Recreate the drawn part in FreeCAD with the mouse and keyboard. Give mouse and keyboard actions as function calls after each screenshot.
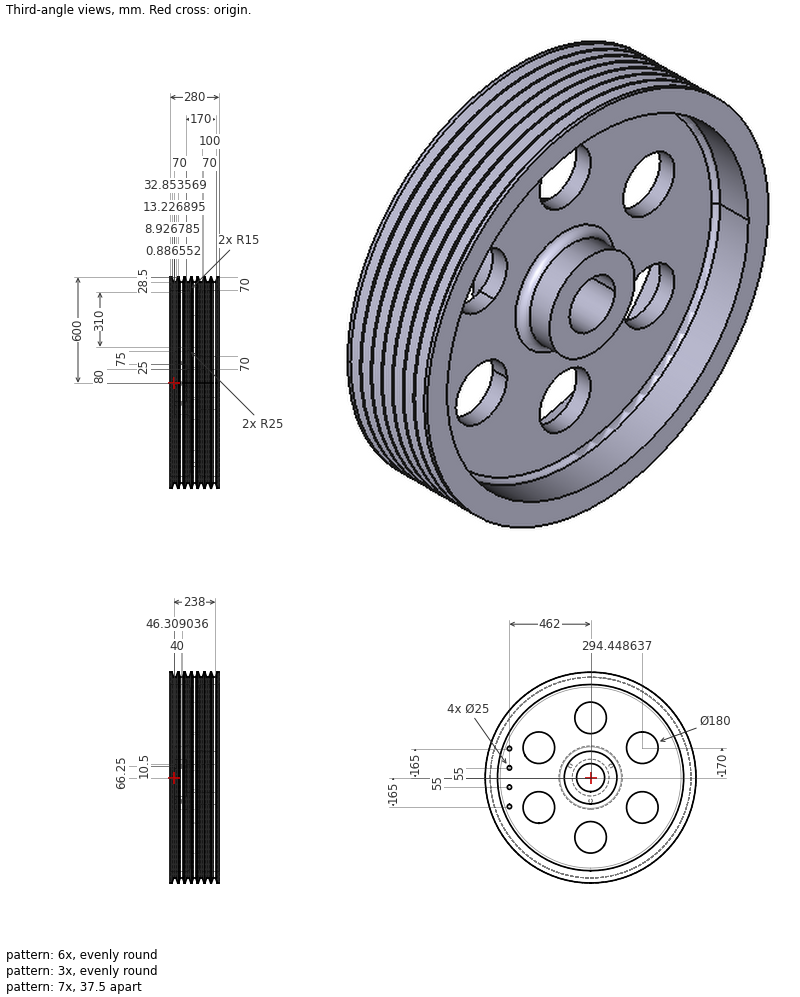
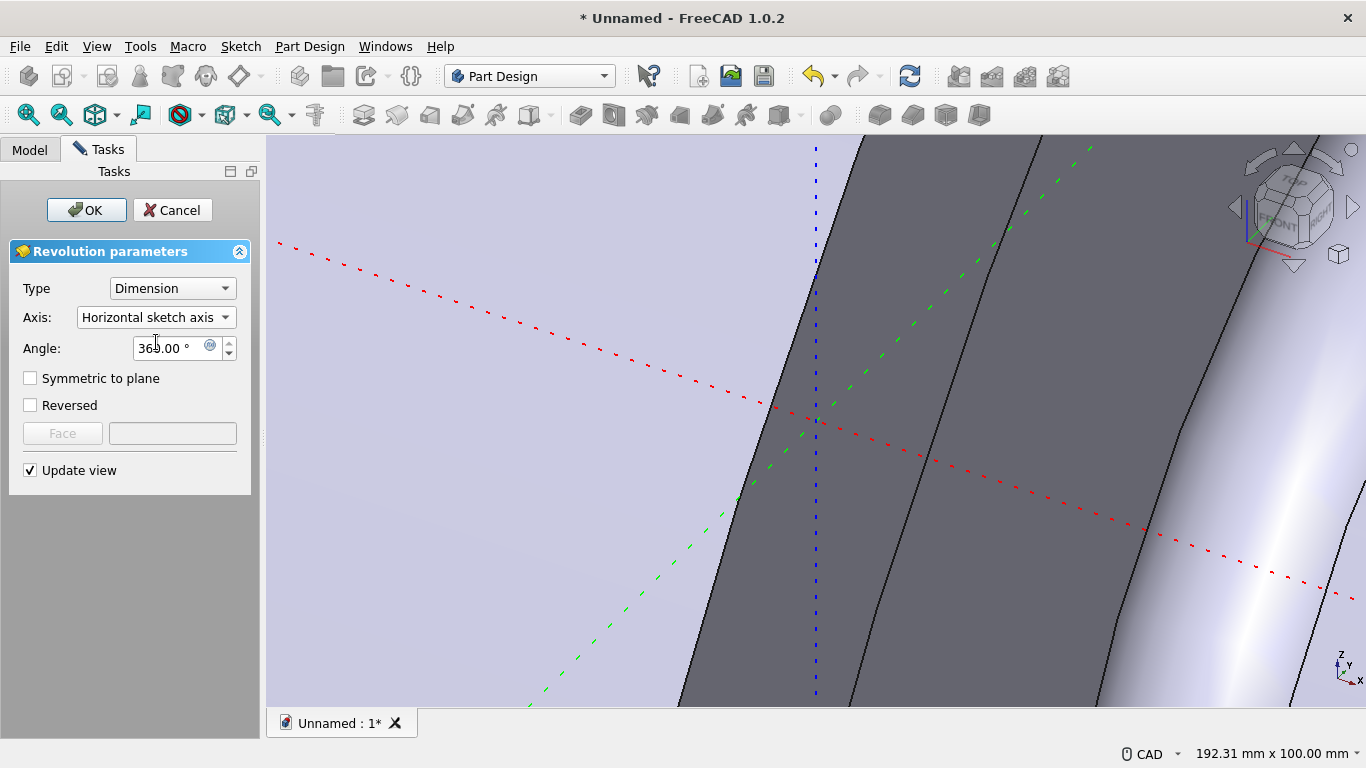
click(87, 210)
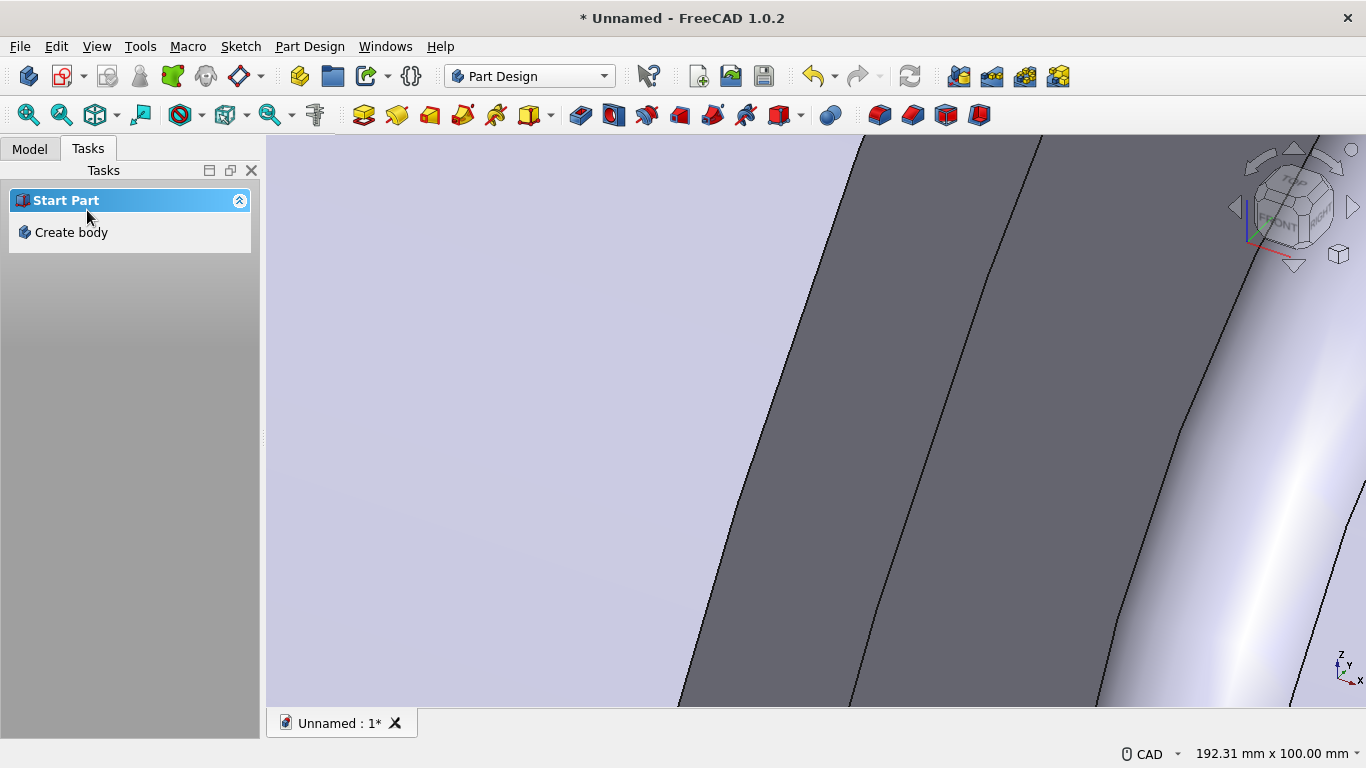
click(29, 116)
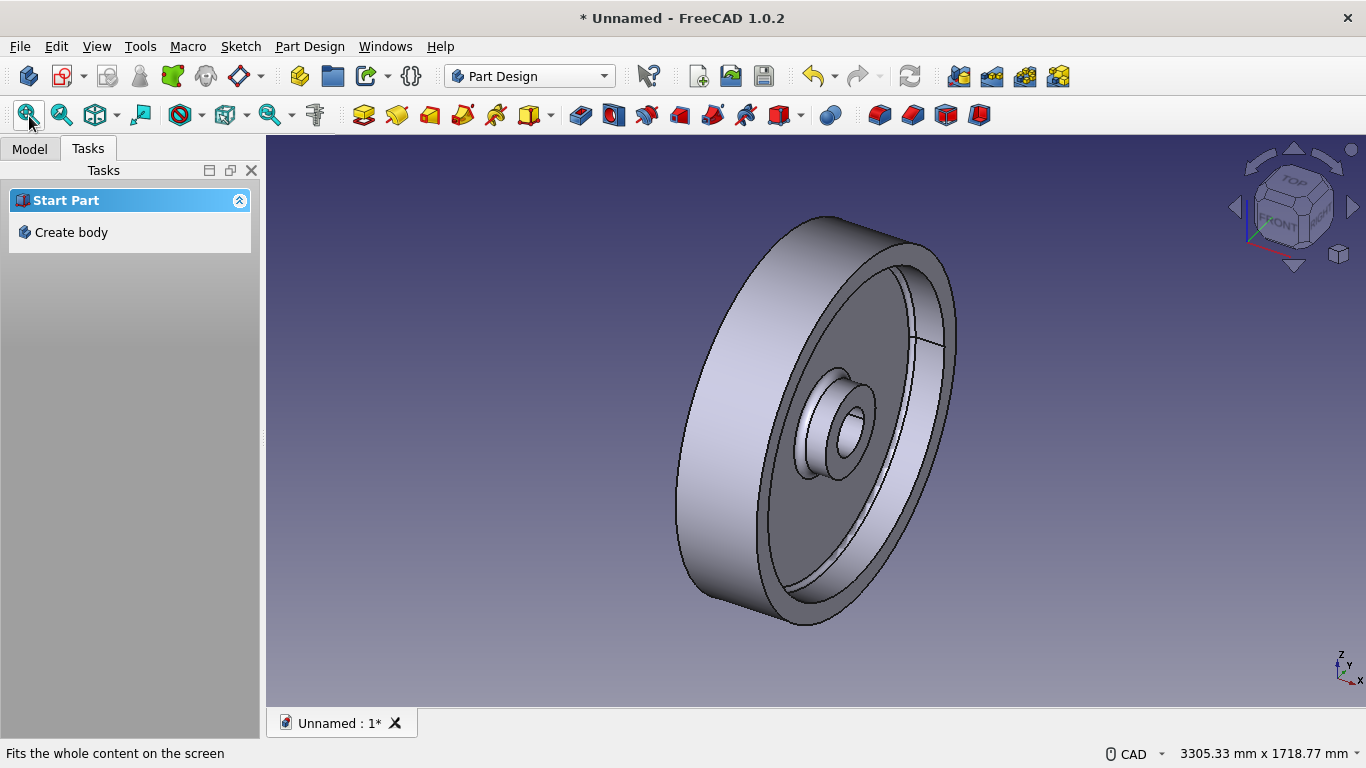
key(6)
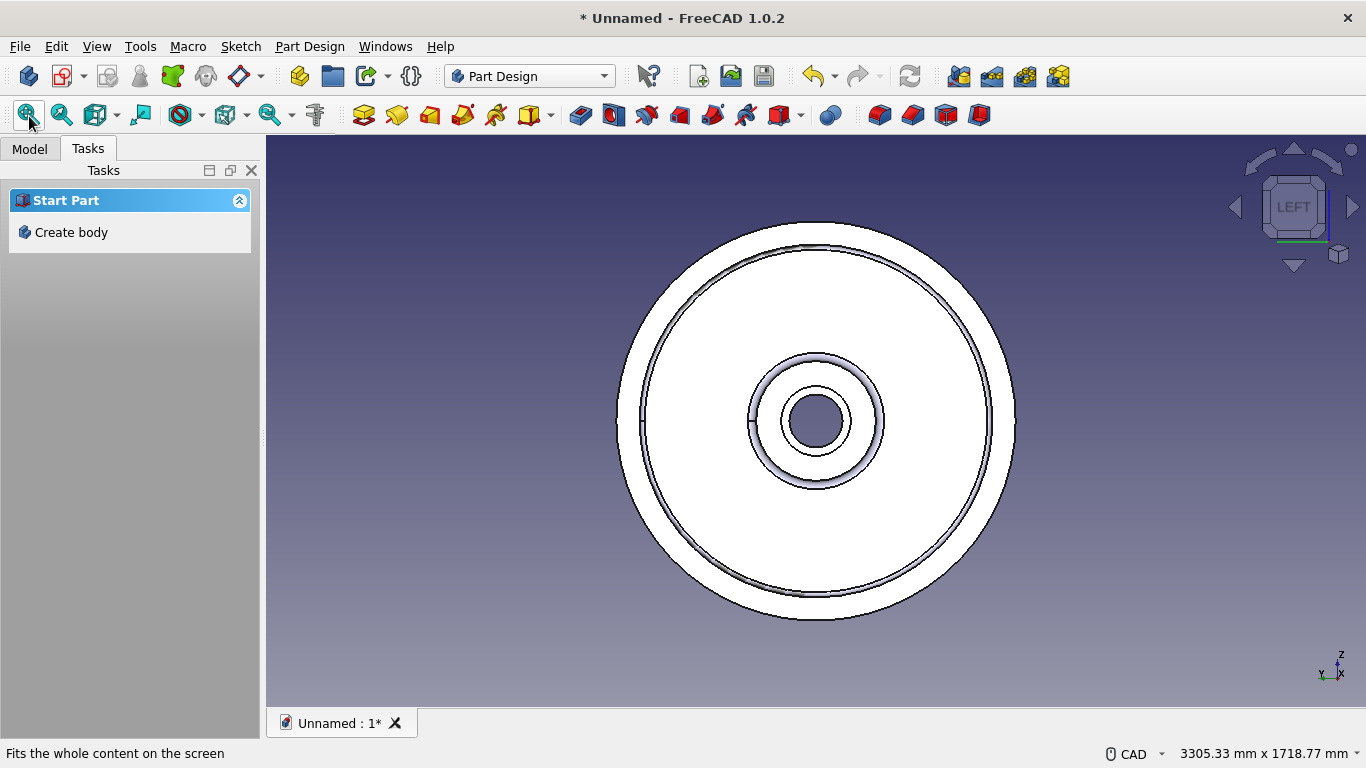
click(782, 386)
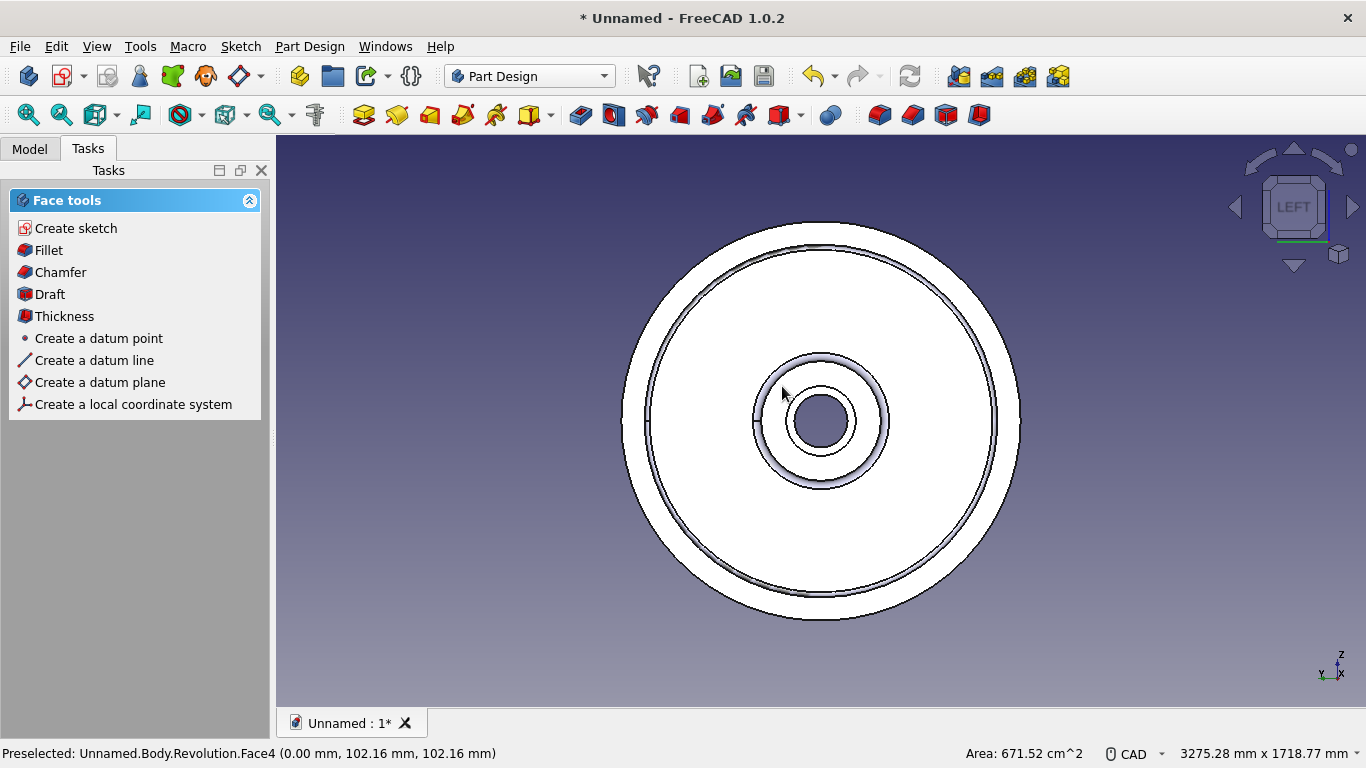
click(62, 76)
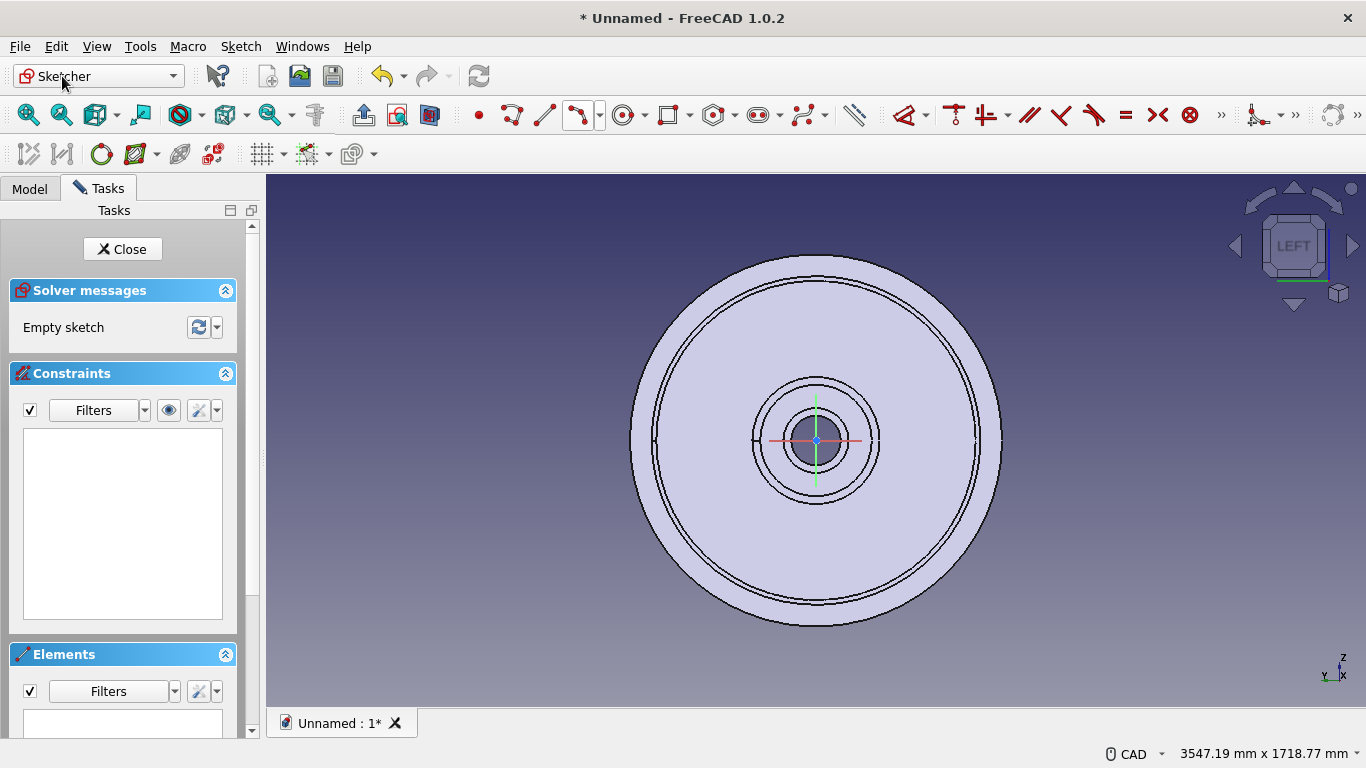
scroll(759, 387, up, 7)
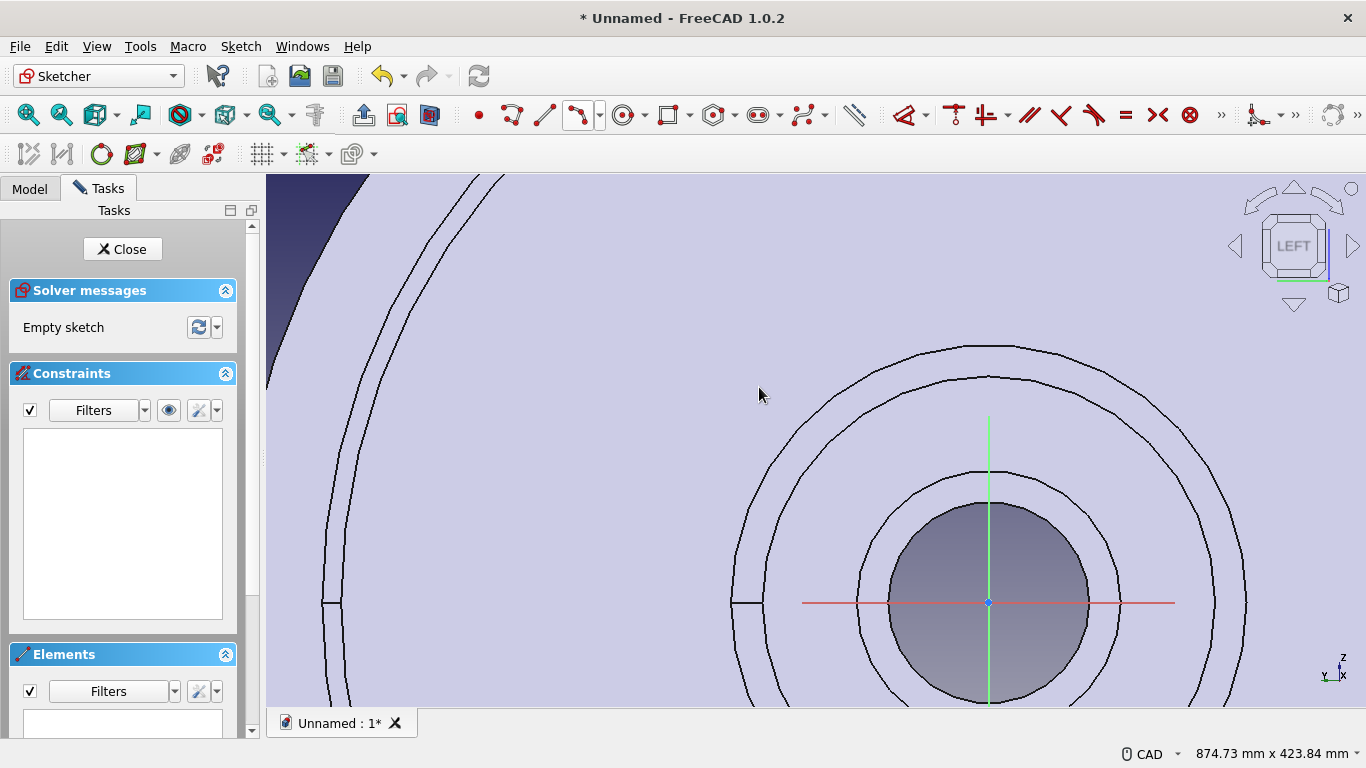
click(622, 116)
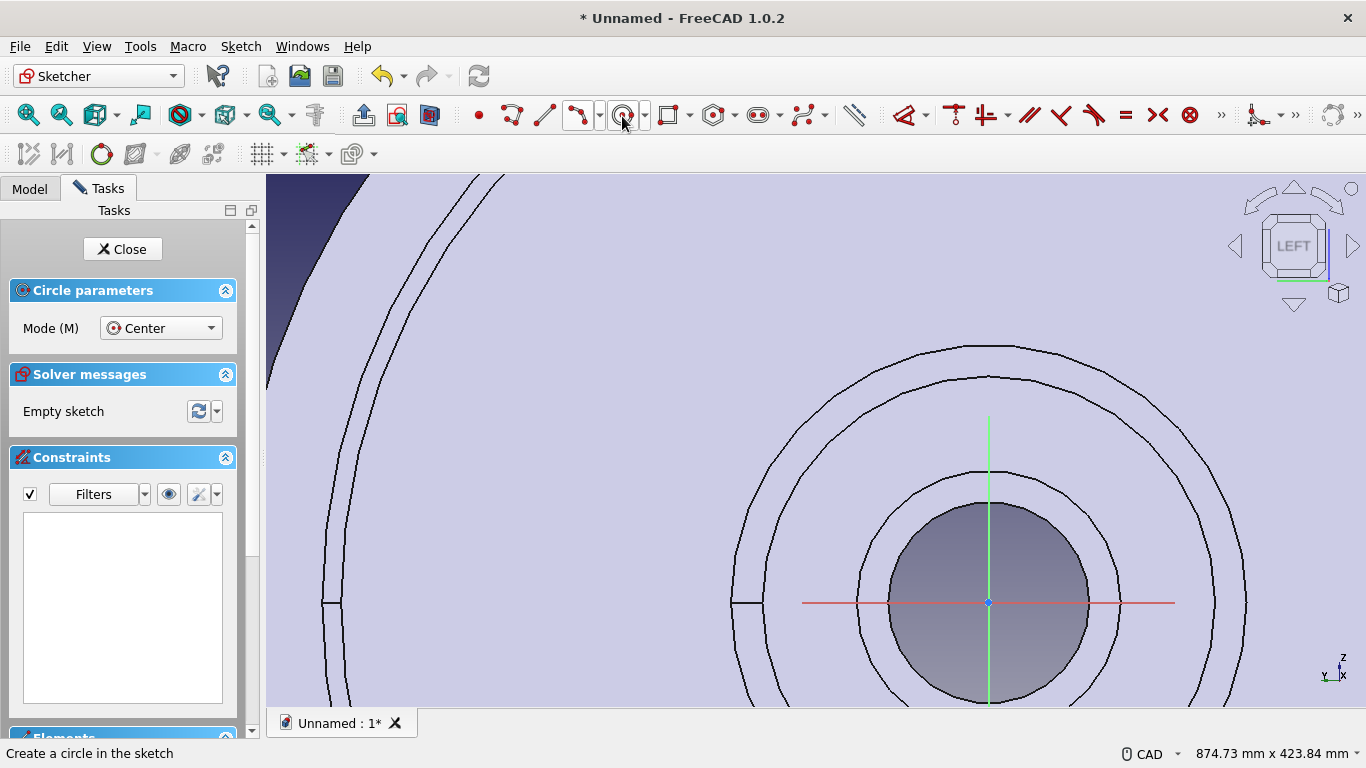
click(618, 389)
move(699, 309)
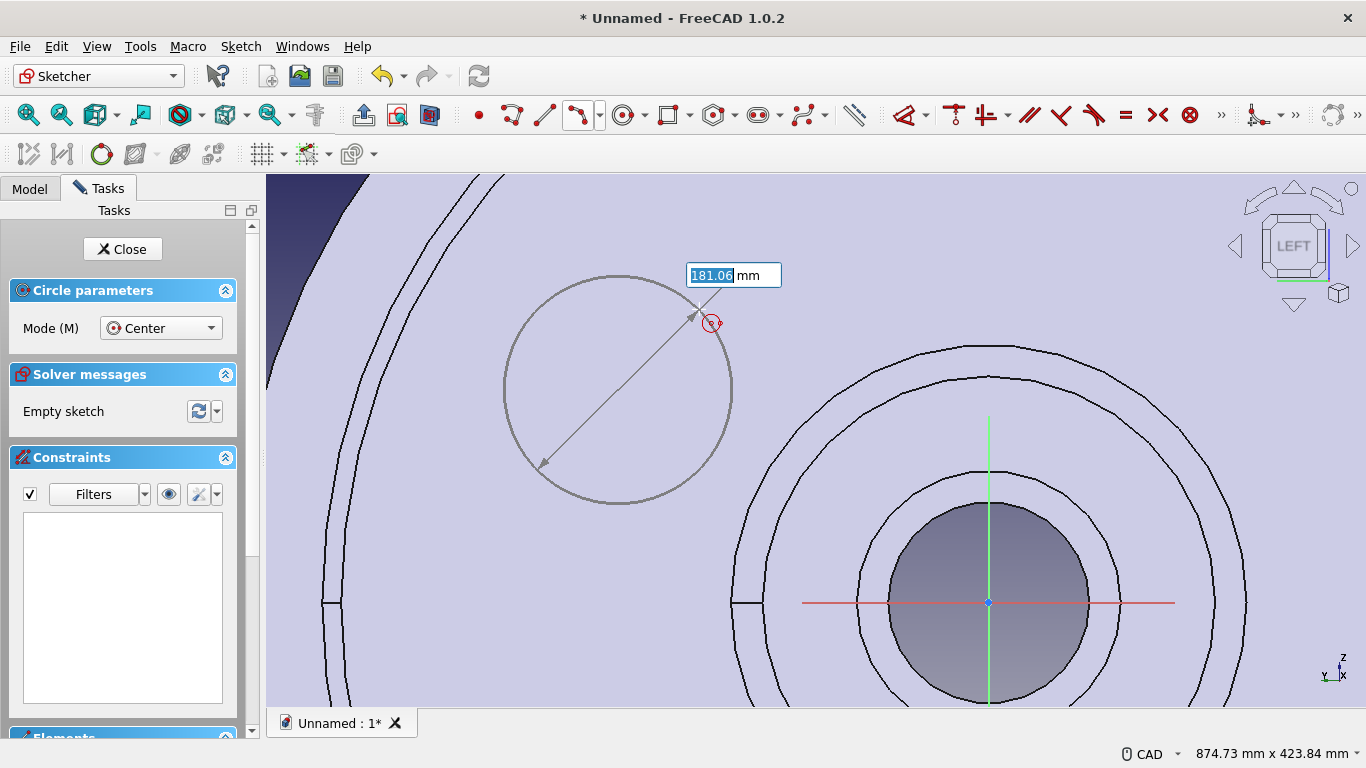
text(180)
key(Return)
key(Escape)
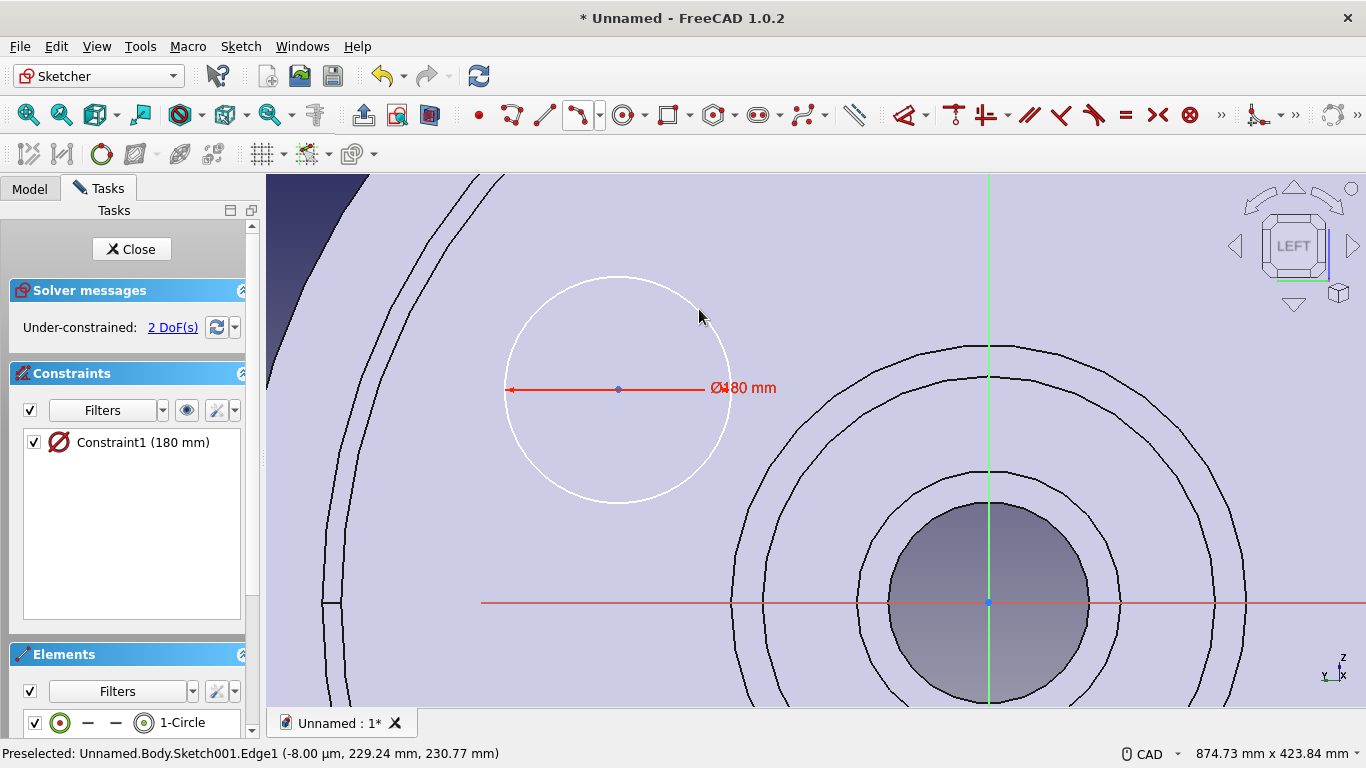
key(d)